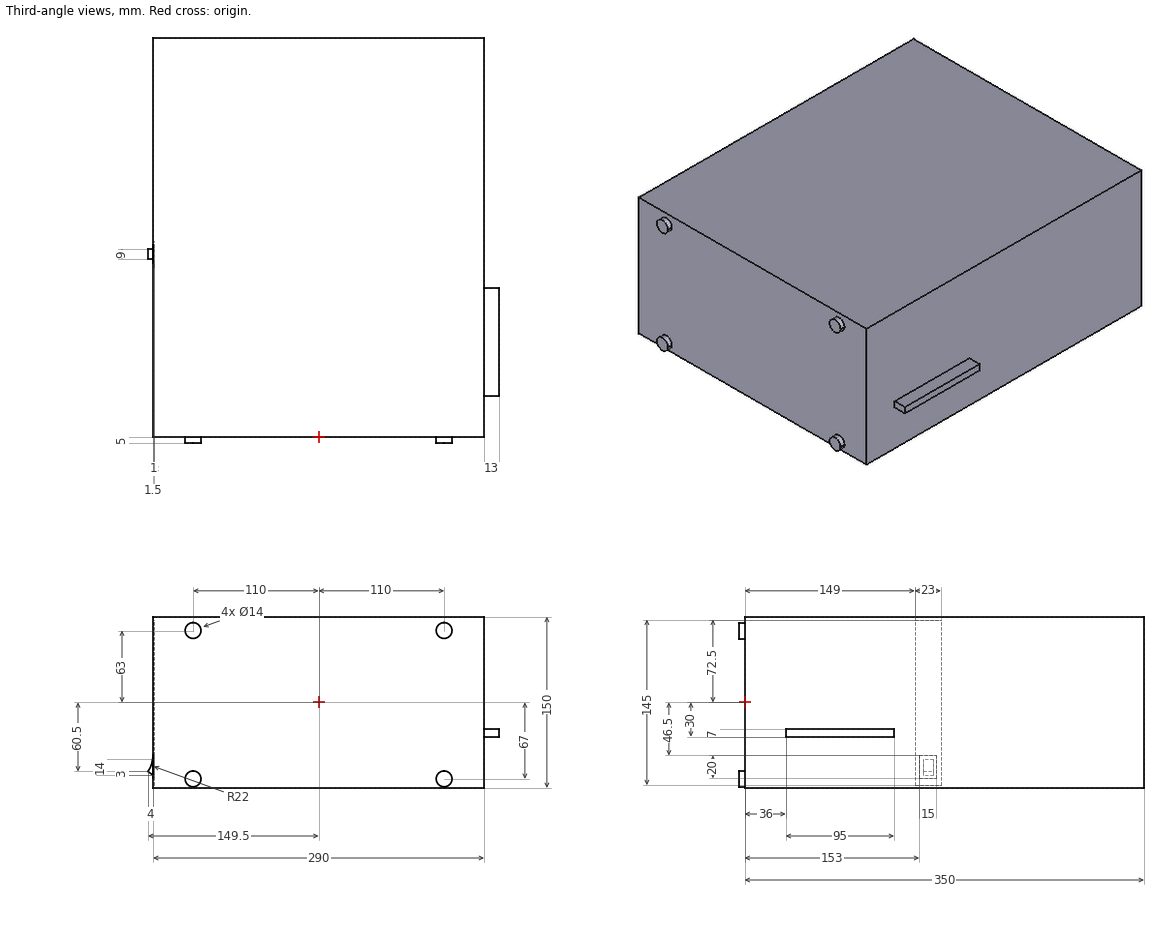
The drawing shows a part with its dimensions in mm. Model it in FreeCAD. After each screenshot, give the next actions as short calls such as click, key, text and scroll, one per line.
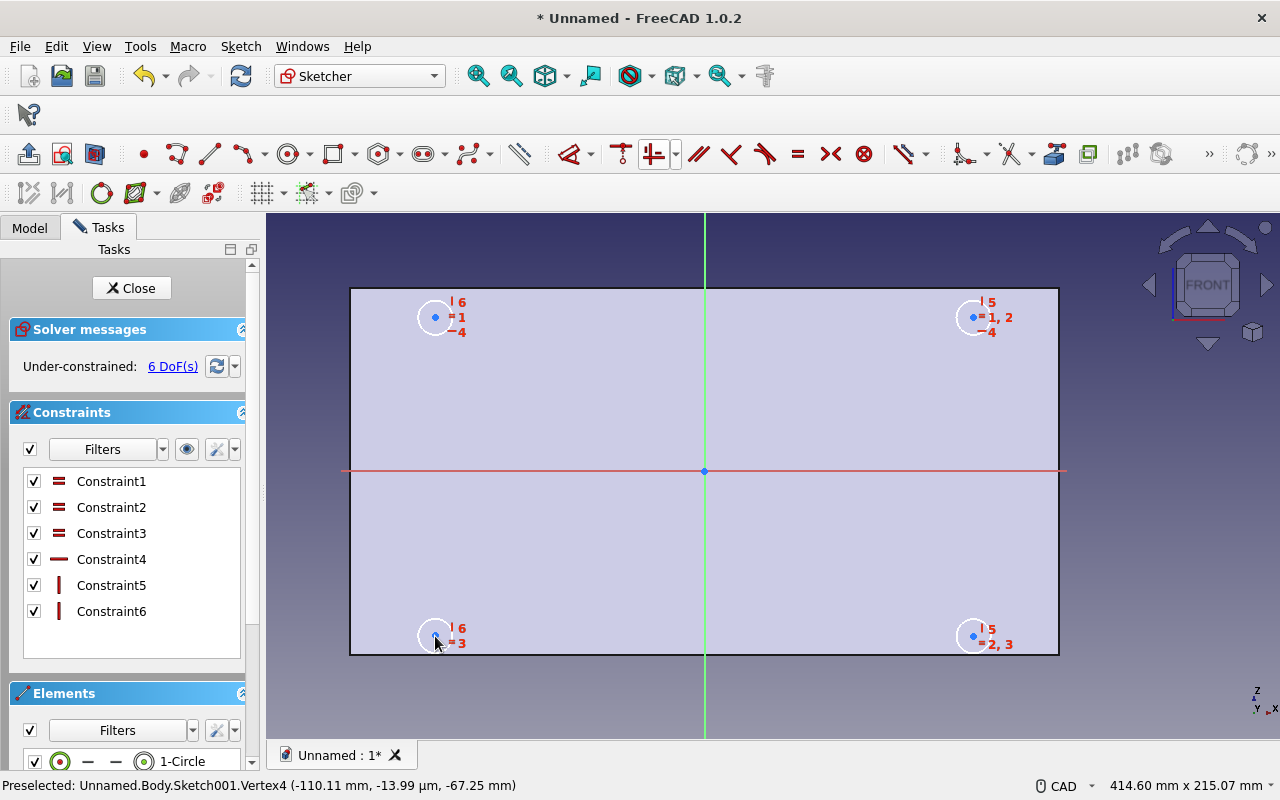
click(974, 636)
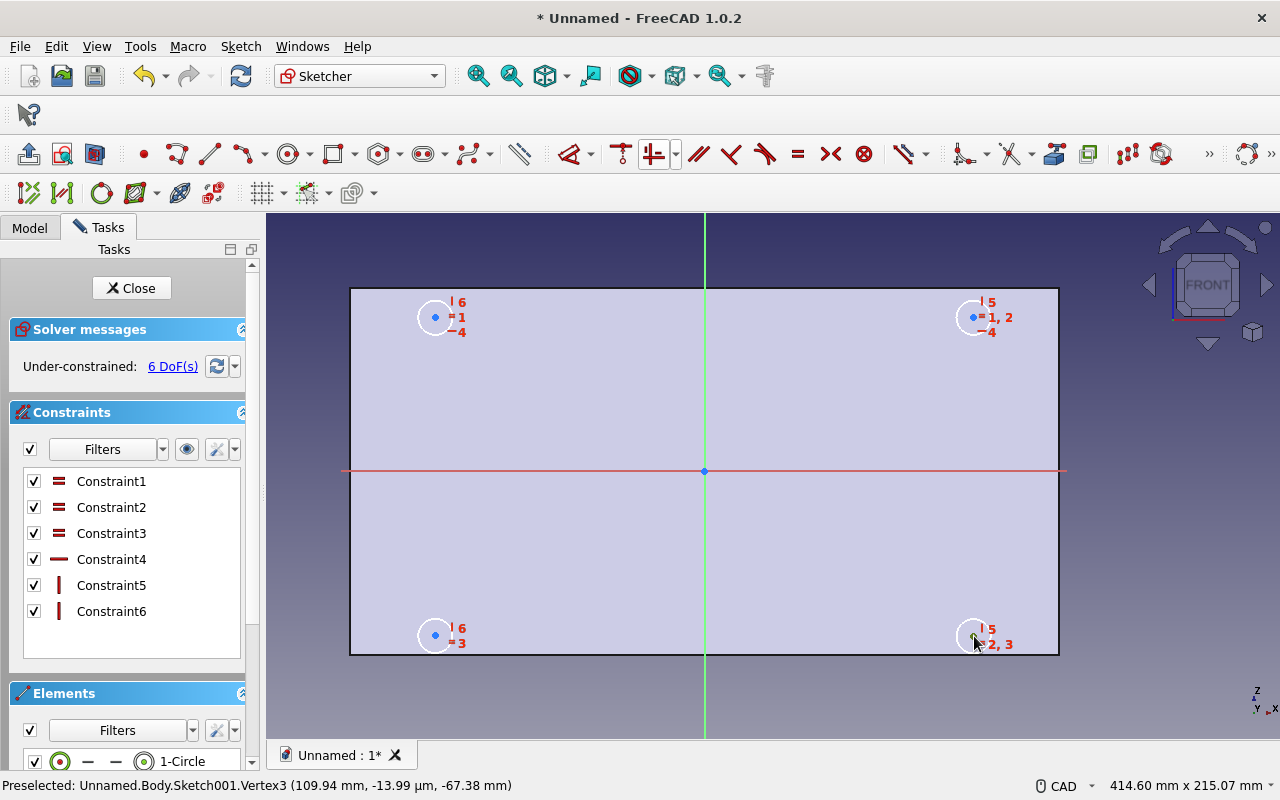
click(435, 636)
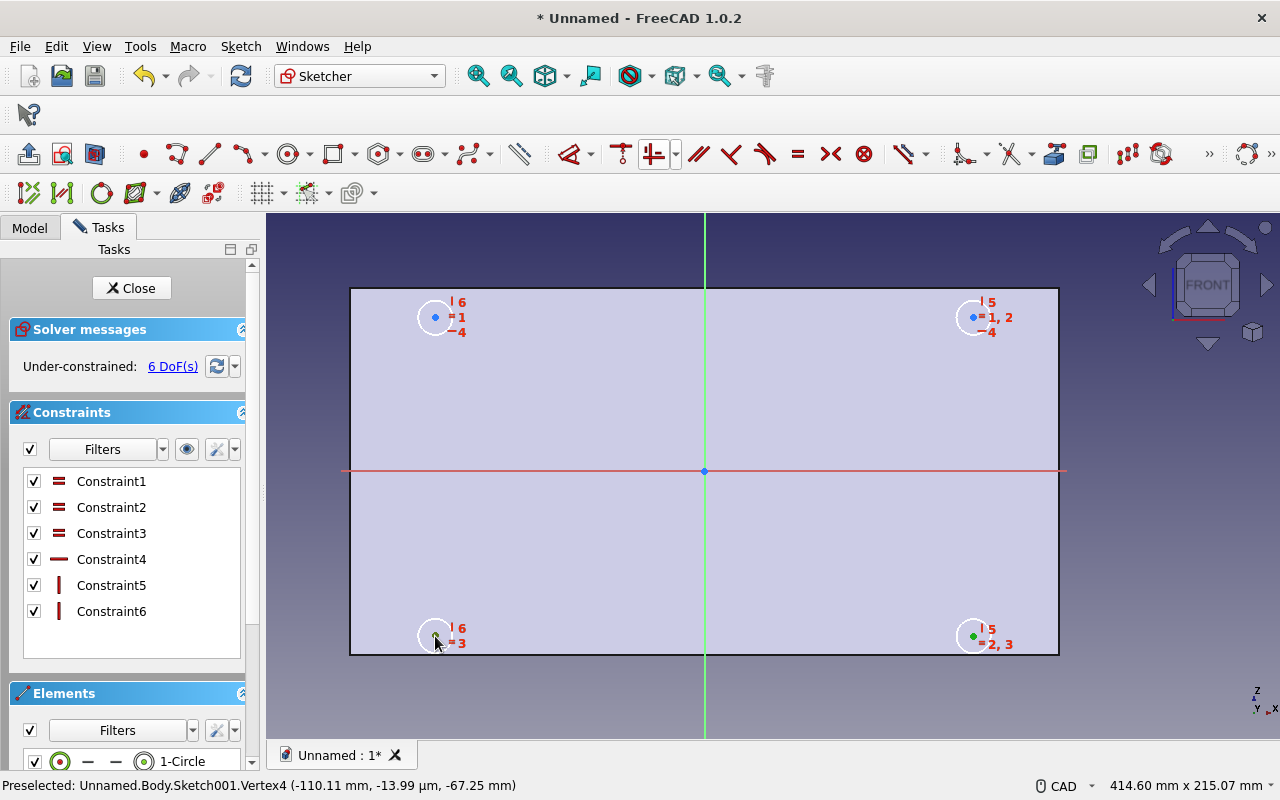
click(676, 154)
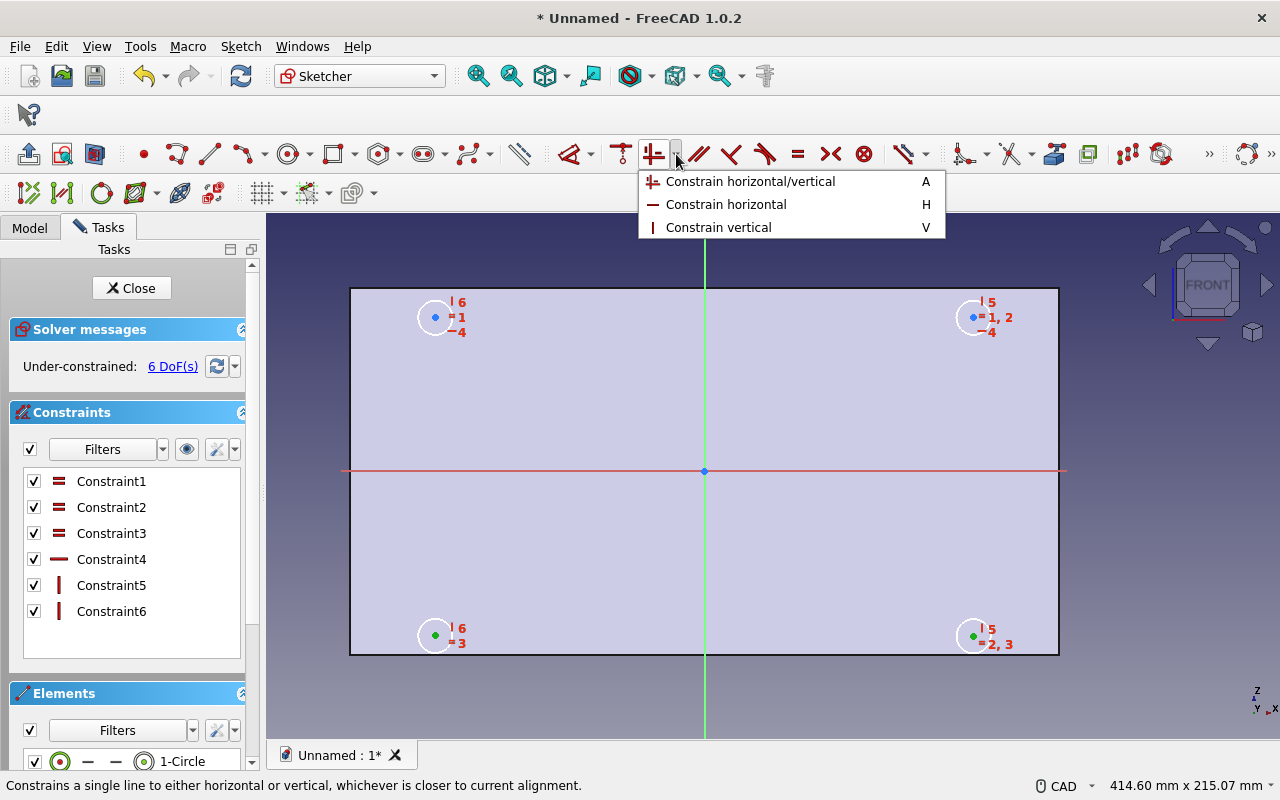
click(792, 204)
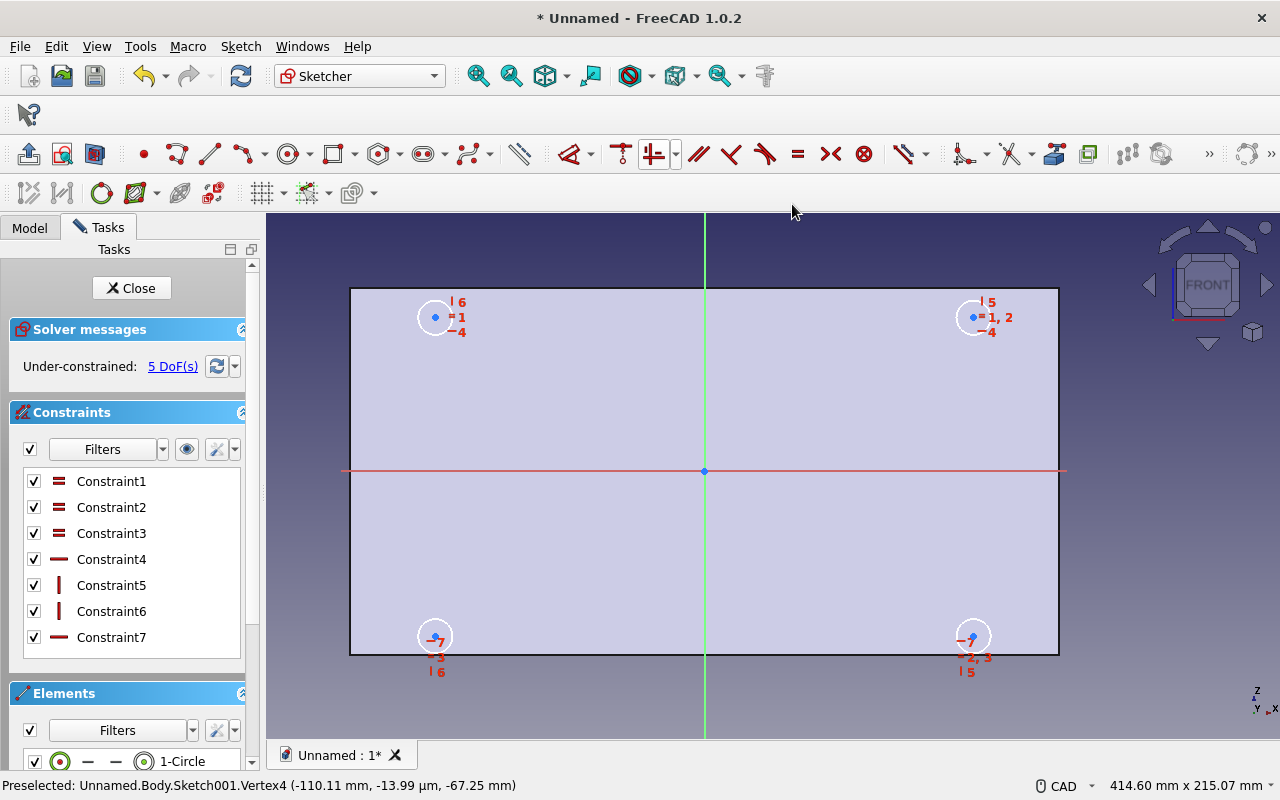
click(568, 154)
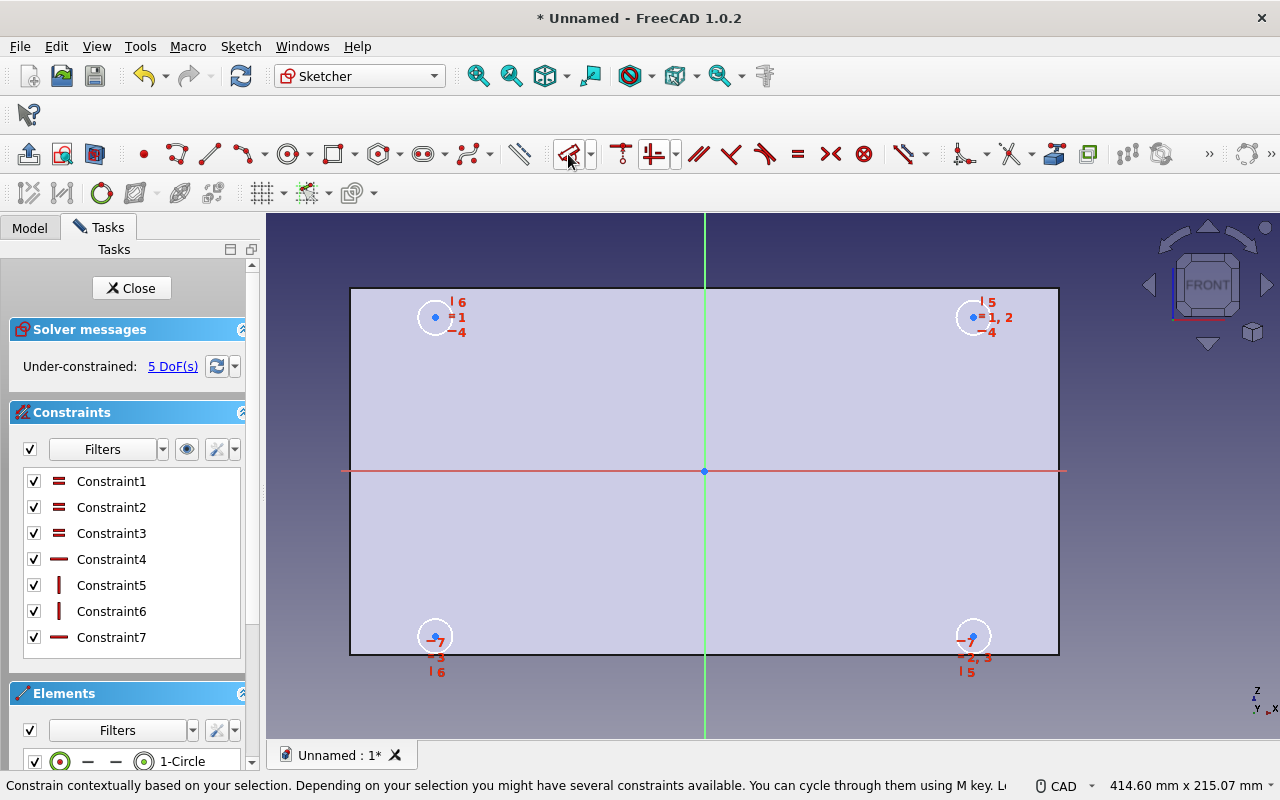
click(447, 306)
click(470, 283)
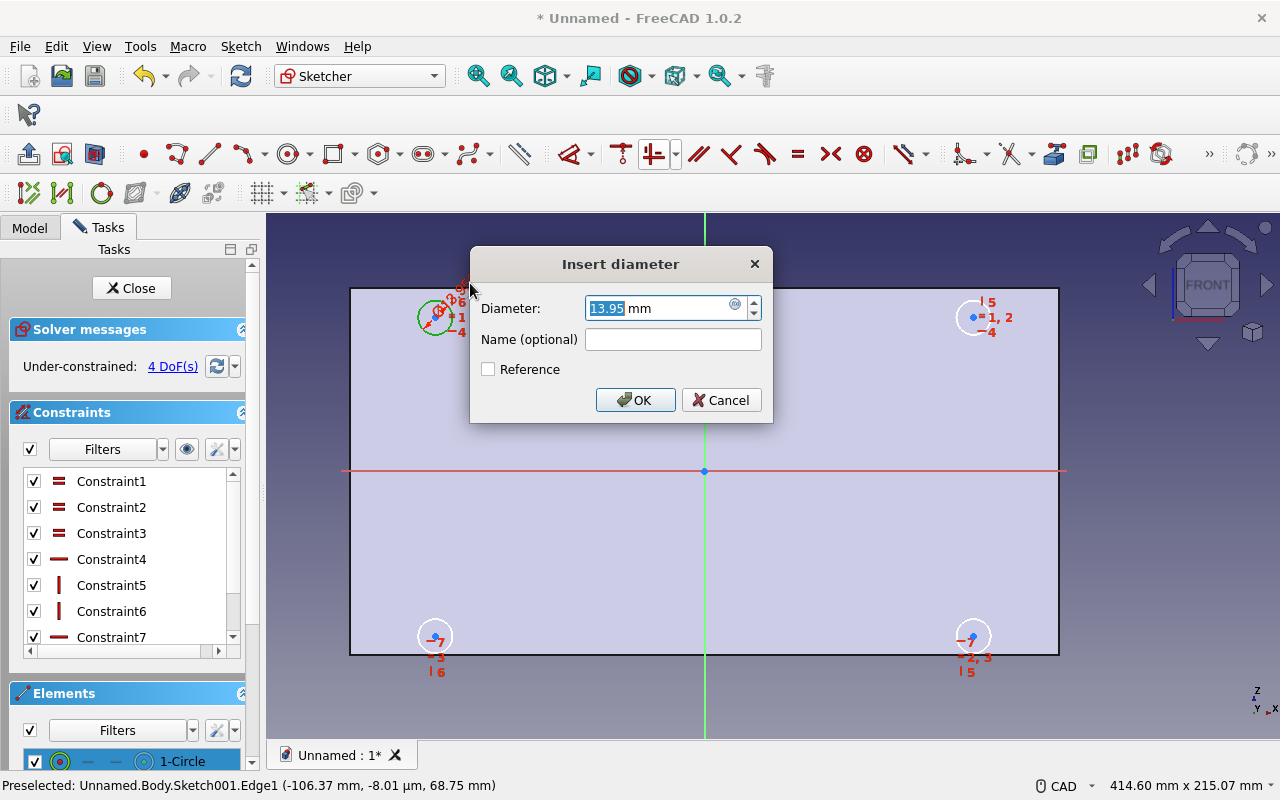
text(14)
key(Return)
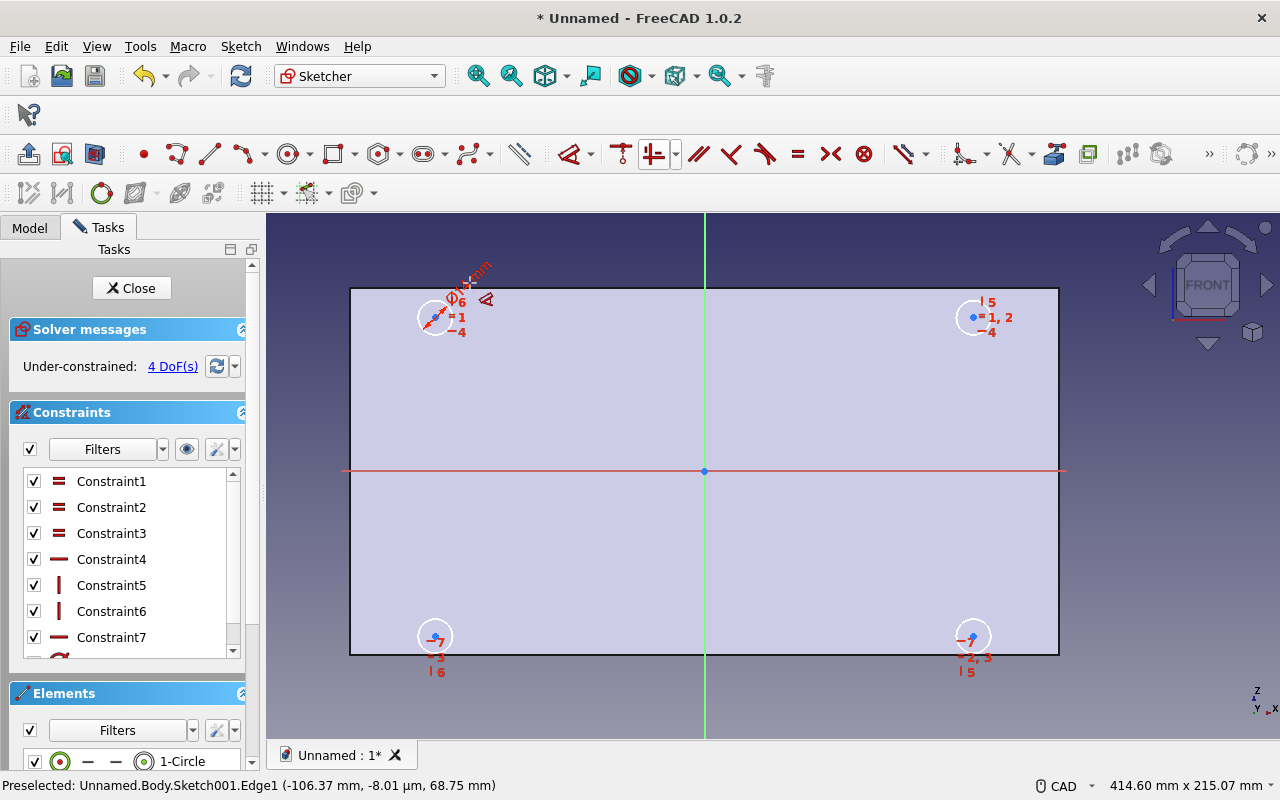
click(435, 318)
click(401, 395)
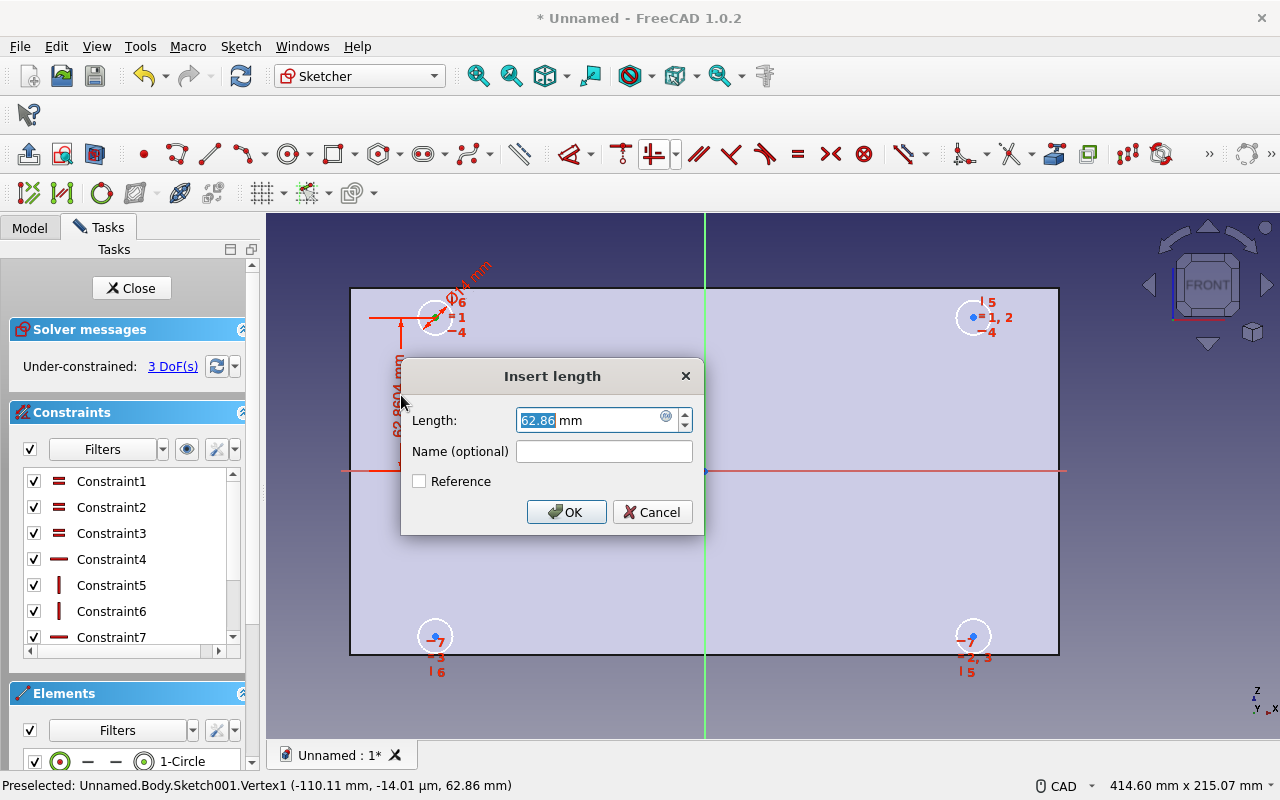
text(63)
key(Return)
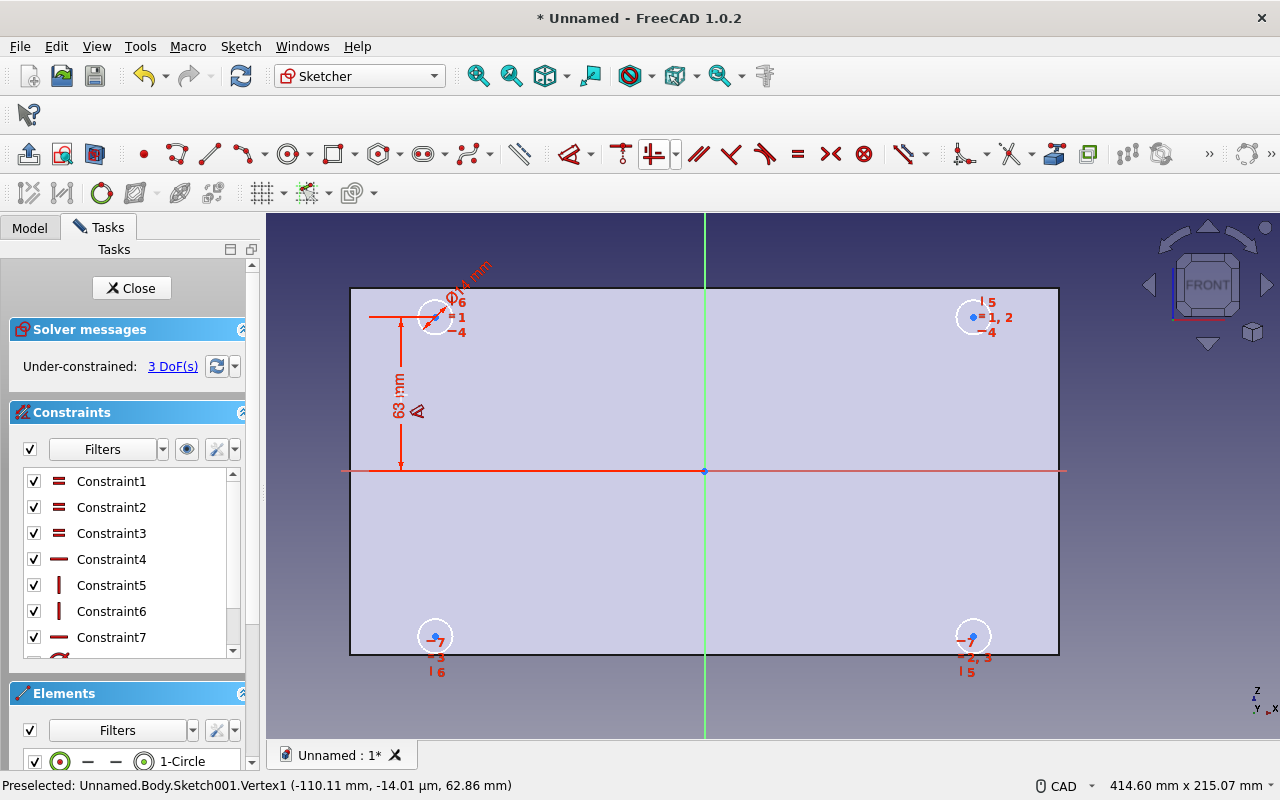
click(974, 636)
click(1008, 554)